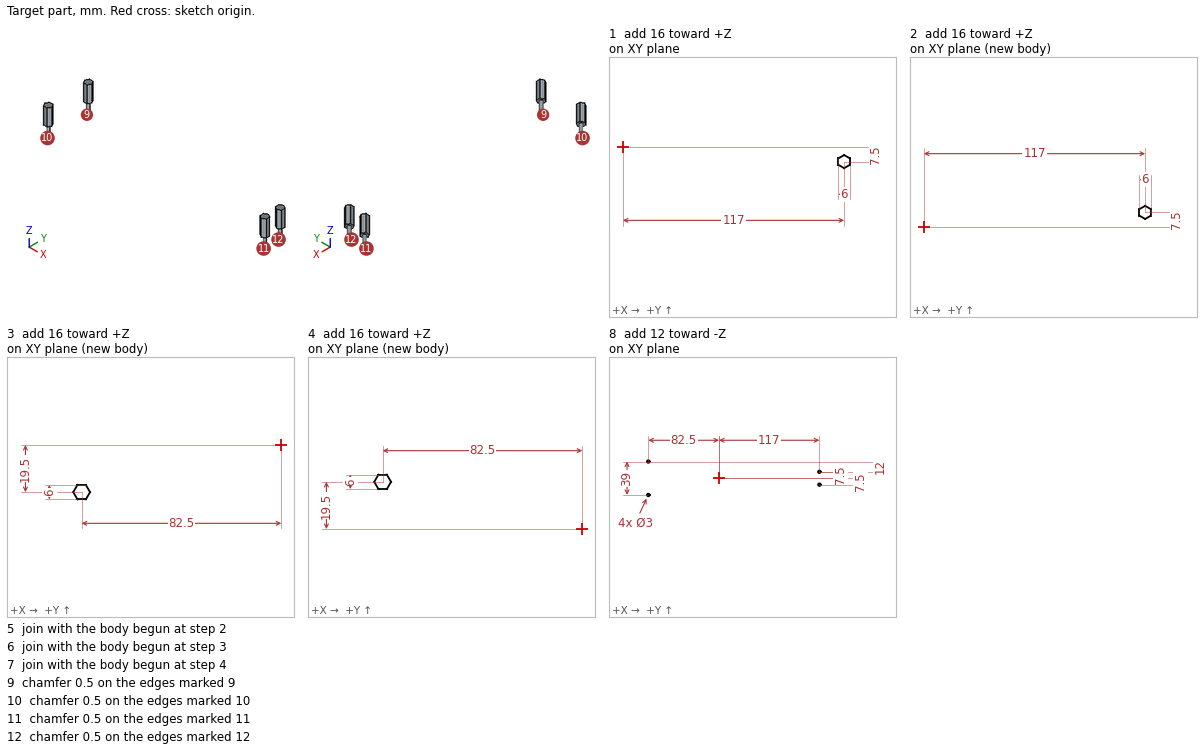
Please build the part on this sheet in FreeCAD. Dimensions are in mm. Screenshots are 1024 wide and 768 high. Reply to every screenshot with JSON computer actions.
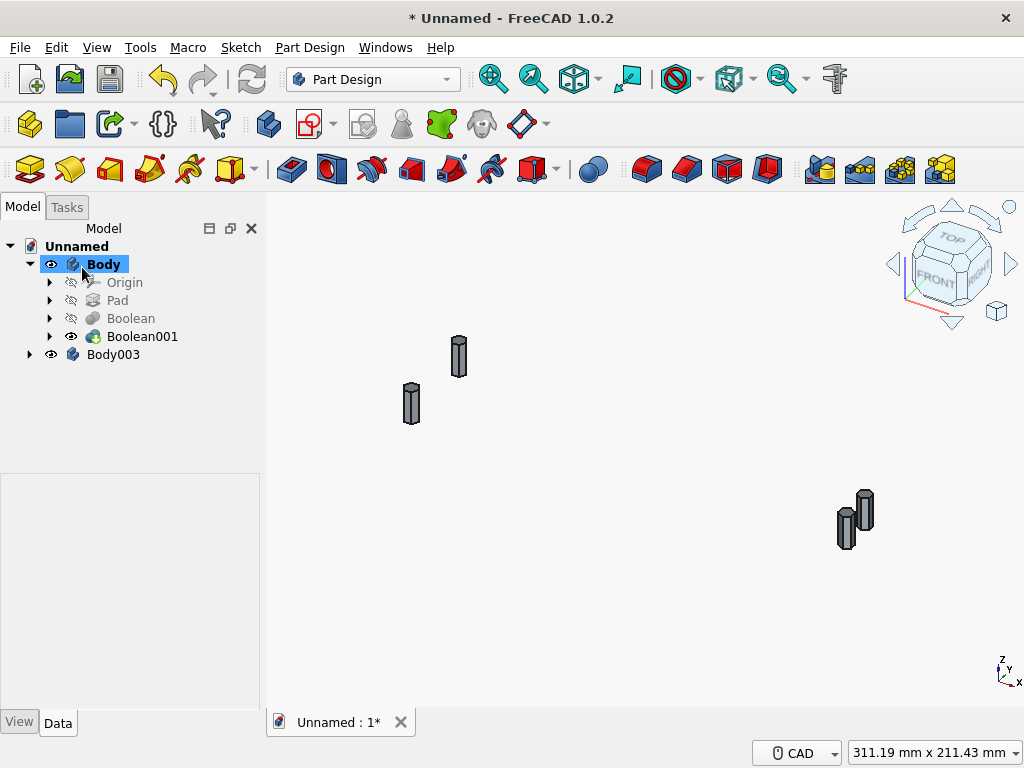
{"action": "left_click", "coordinate": [96, 354]}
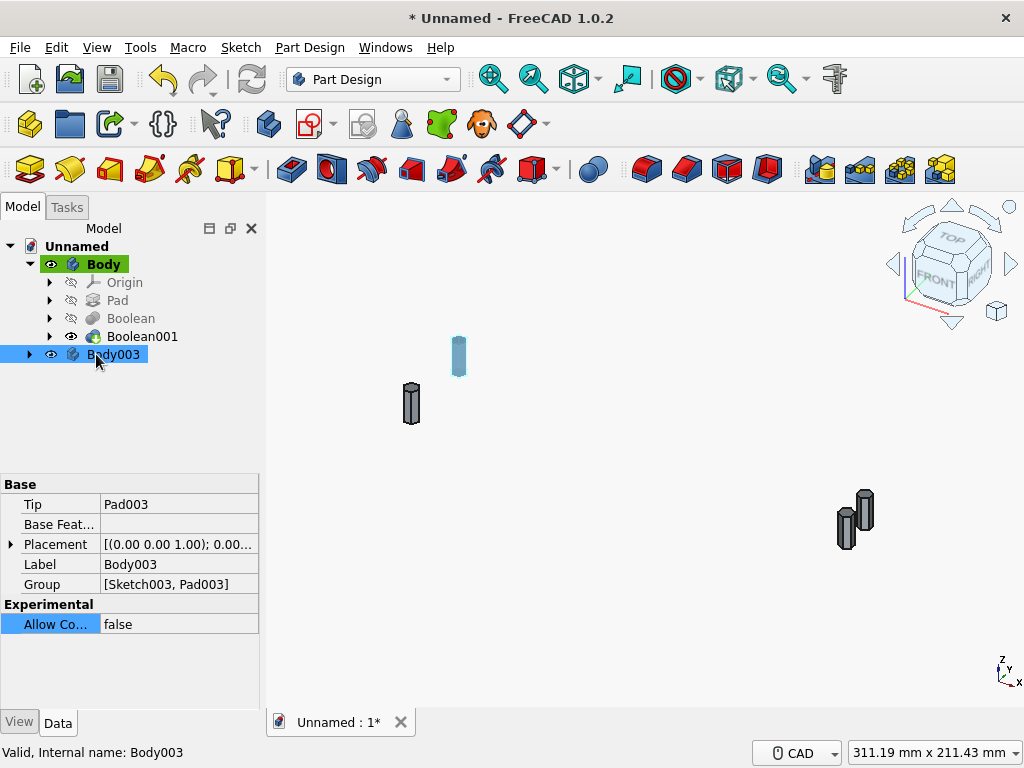
{"action": "left_click", "coordinate": [594, 170]}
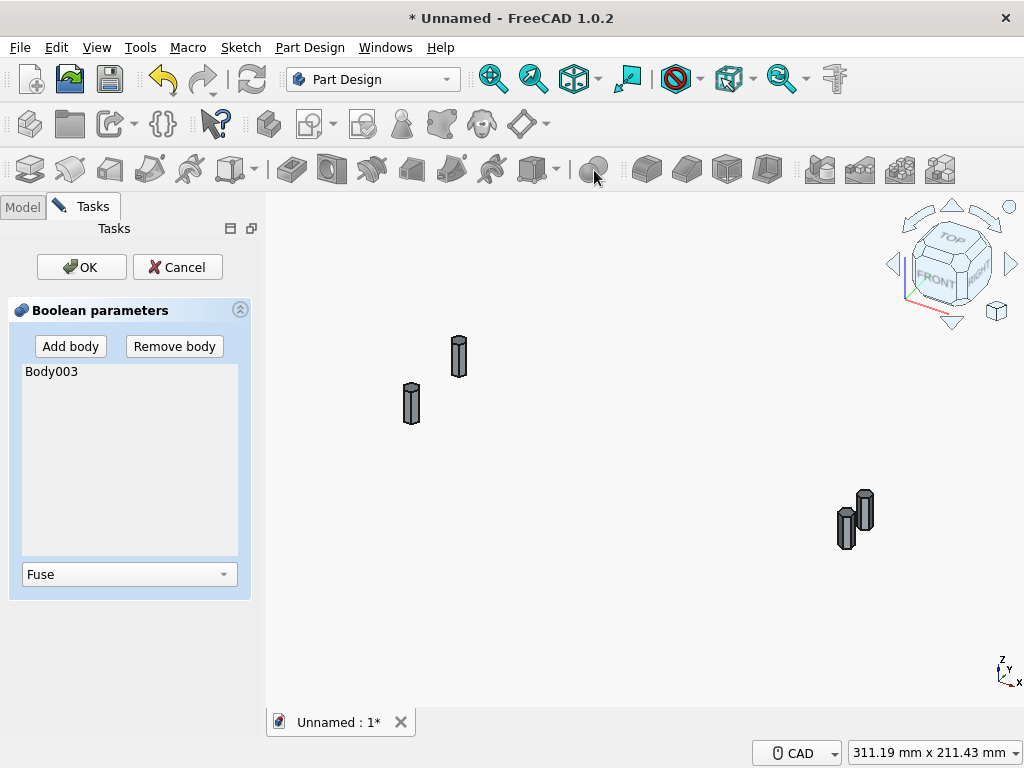
{"action": "left_click", "coordinate": [82, 267]}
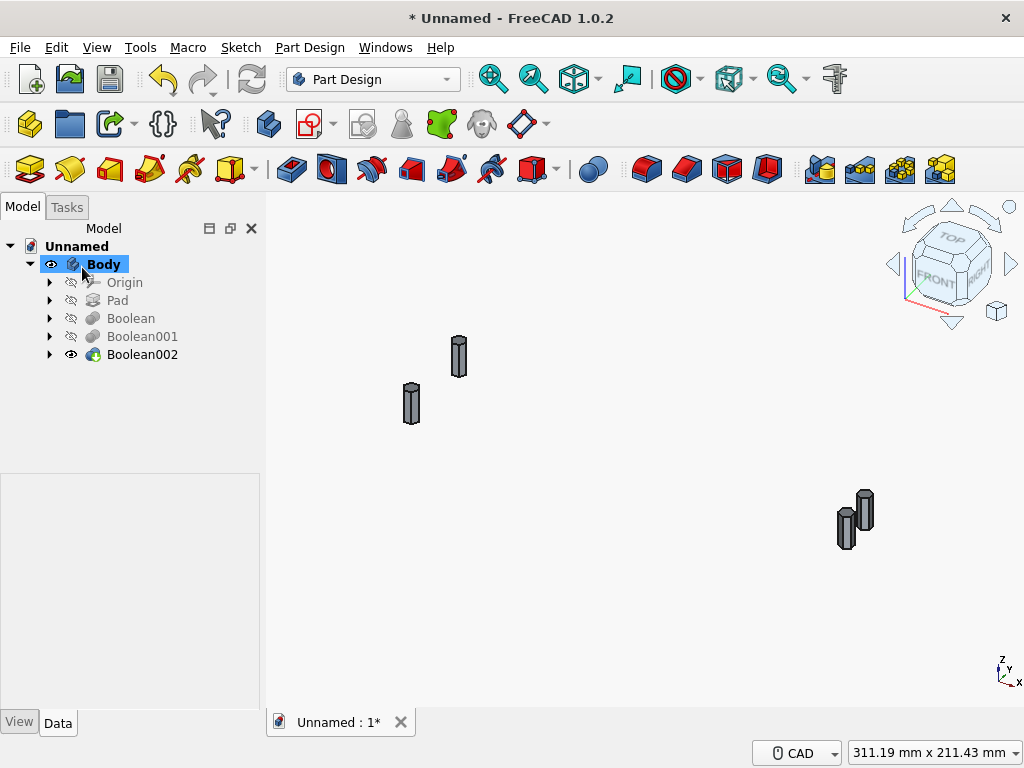
{"action": "key", "text": "5"}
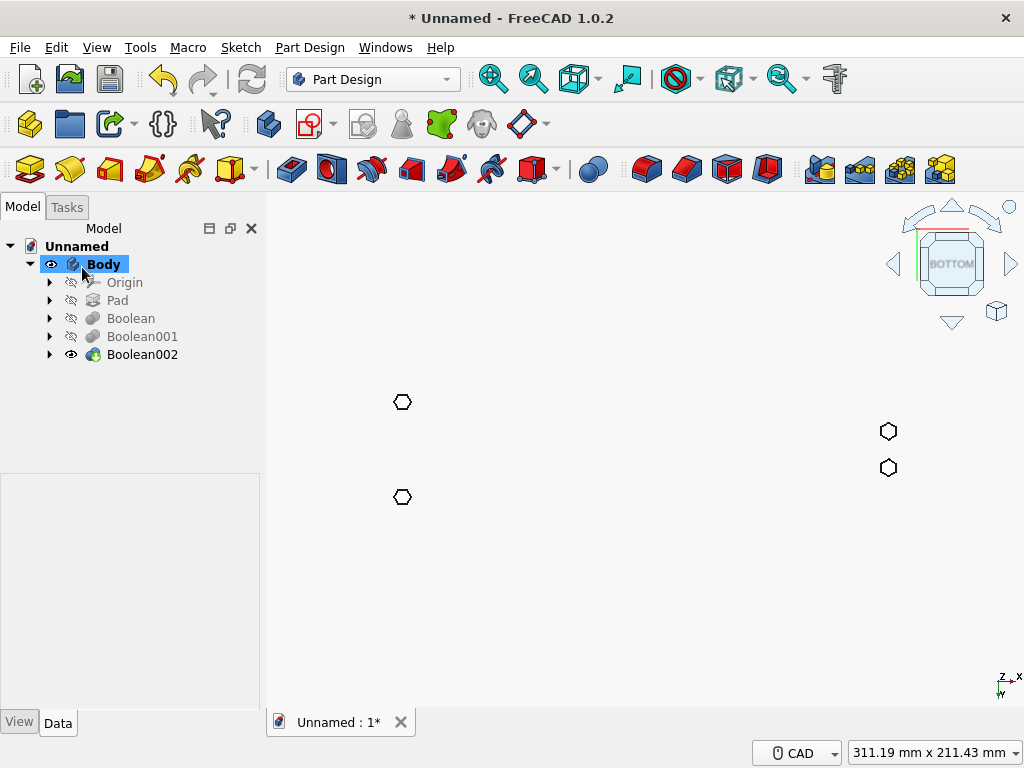
{"action": "key", "text": "1"}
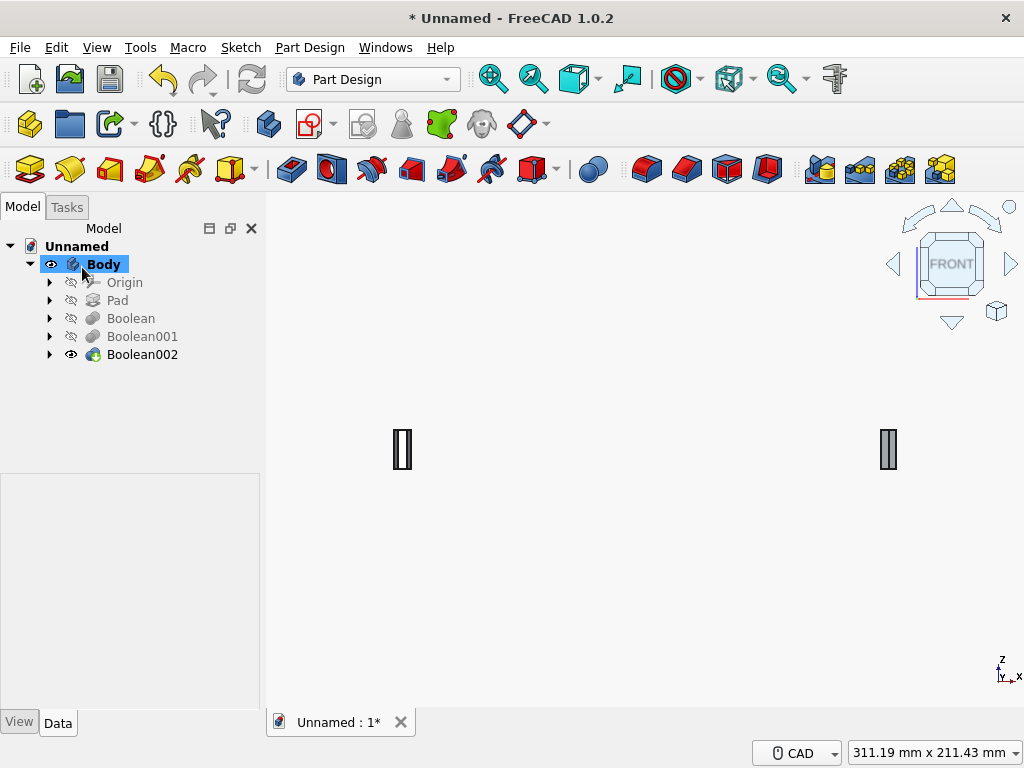
{"action": "key", "text": "3"}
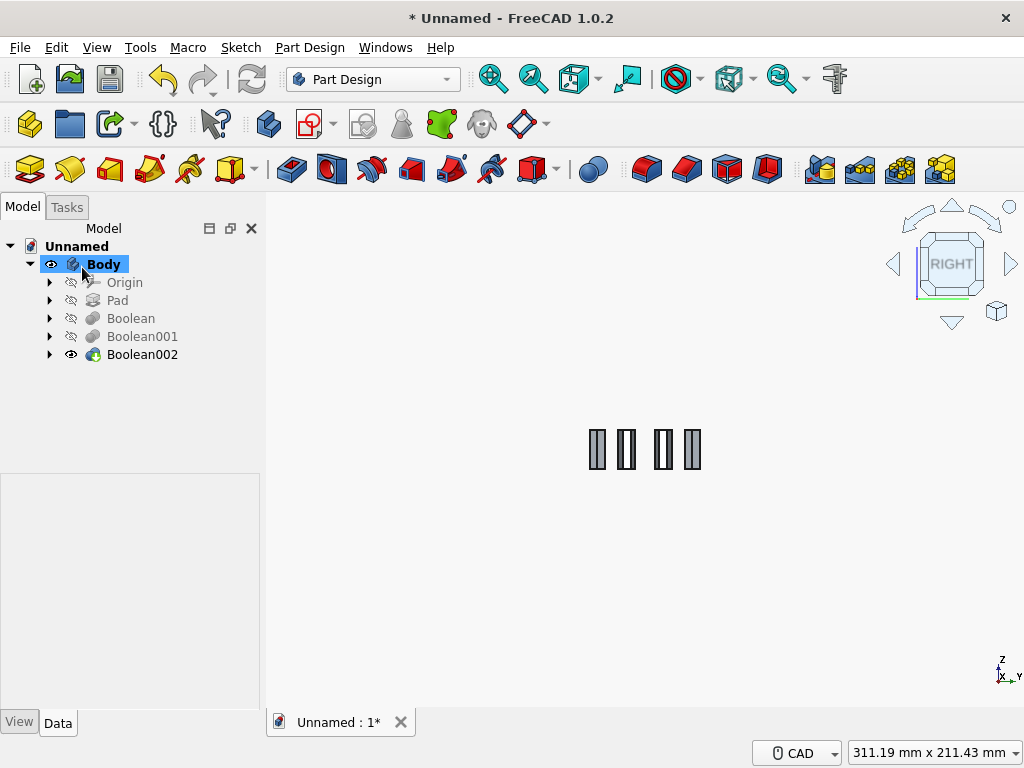
{"action": "left_click", "coordinate": [494, 80]}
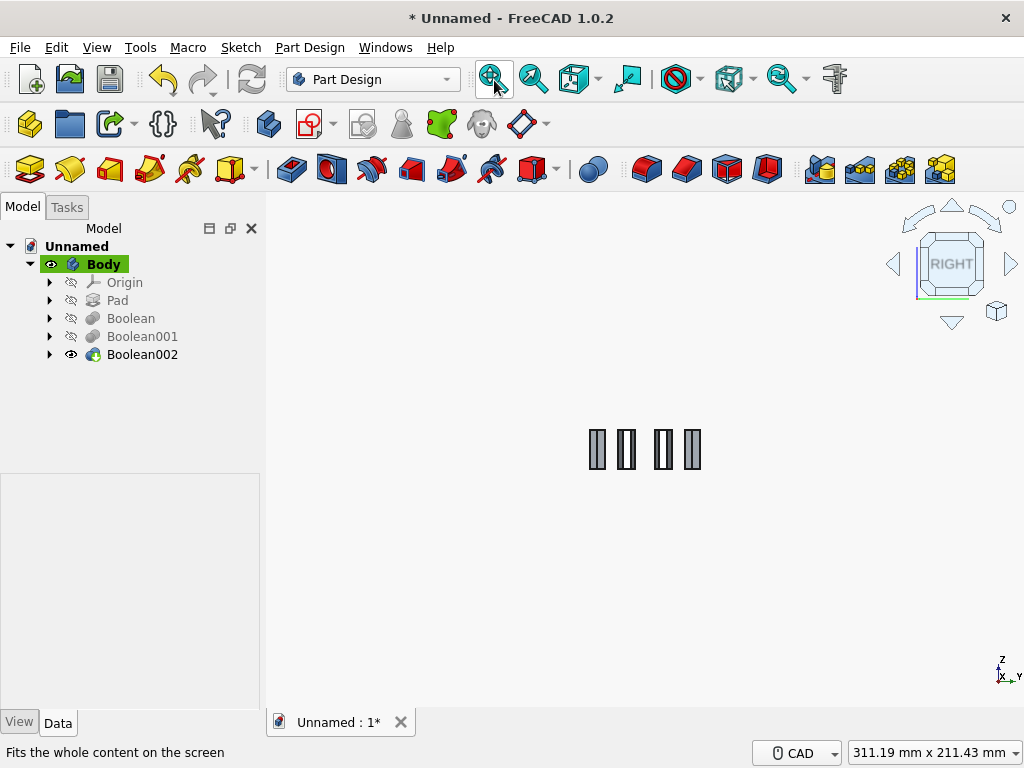
{"action": "left_click", "coordinate": [310, 124]}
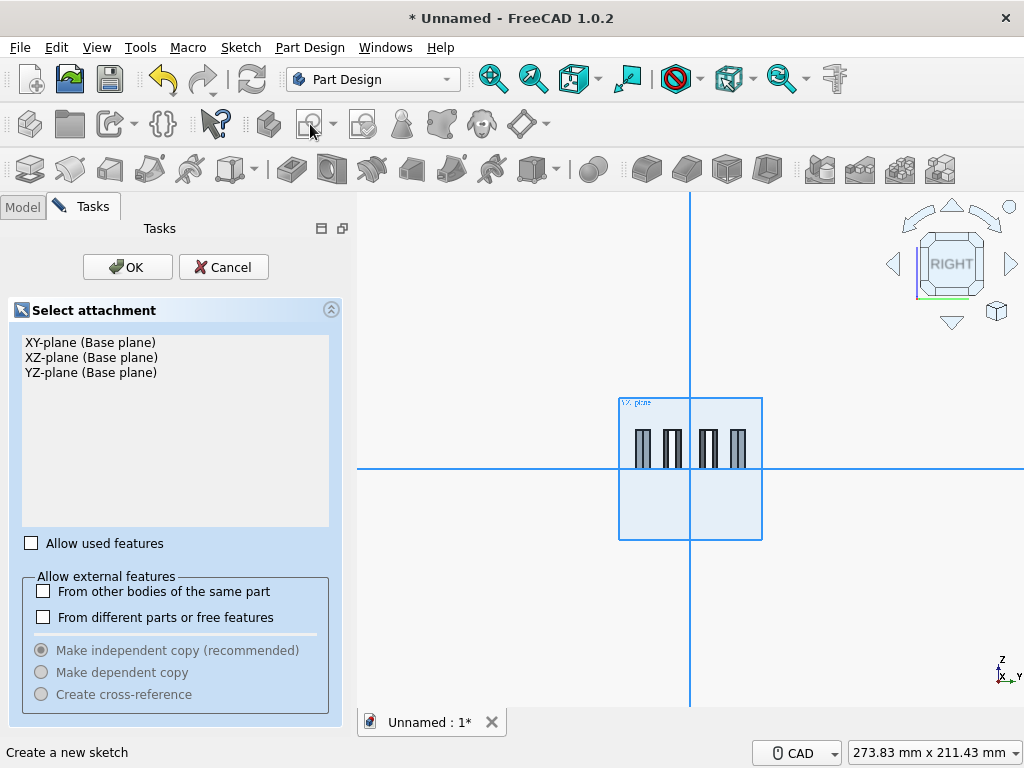
{"action": "left_click", "coordinate": [82, 342]}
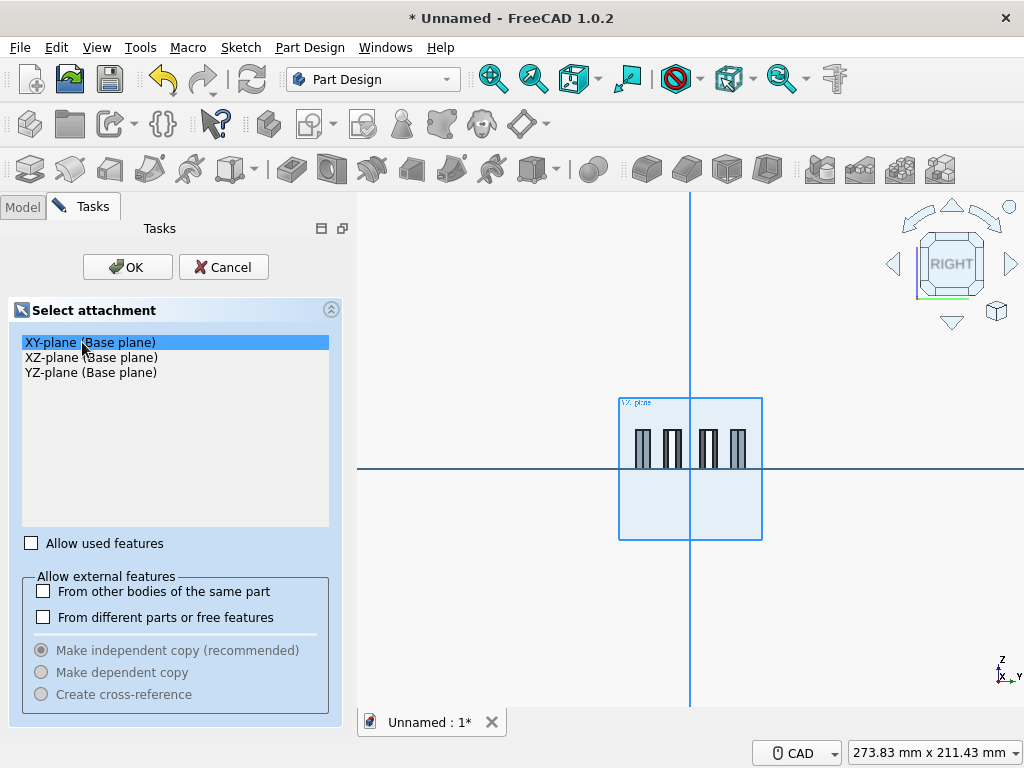
{"action": "left_click", "coordinate": [128, 267]}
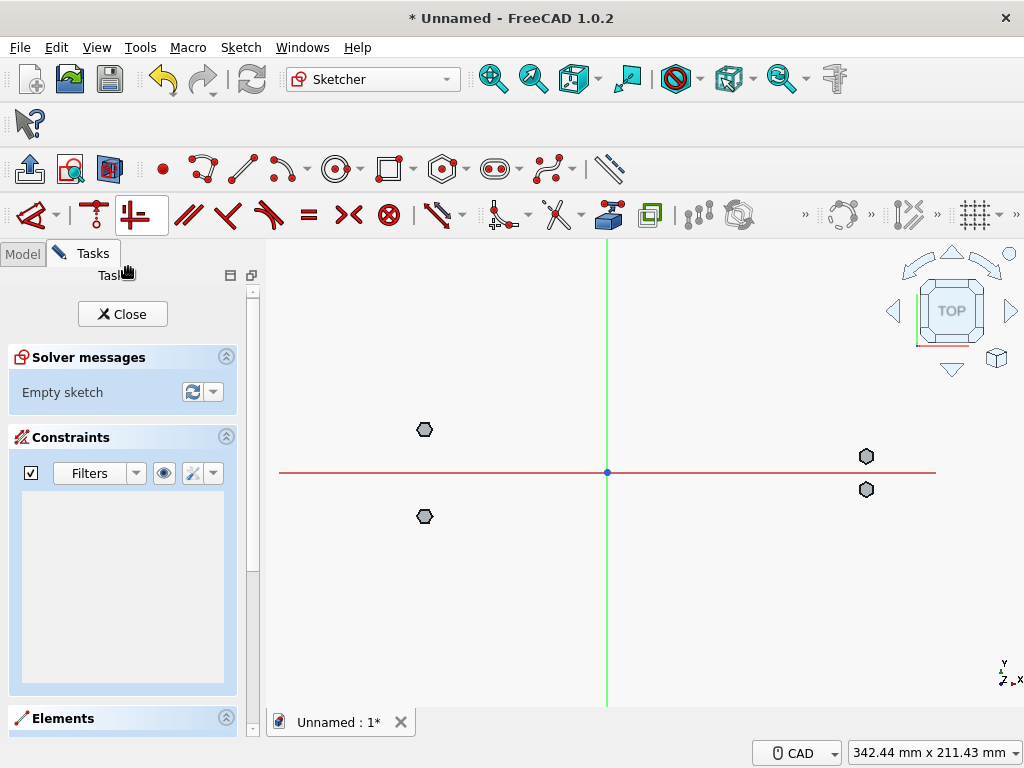
{"action": "left_click", "coordinate": [110, 170]}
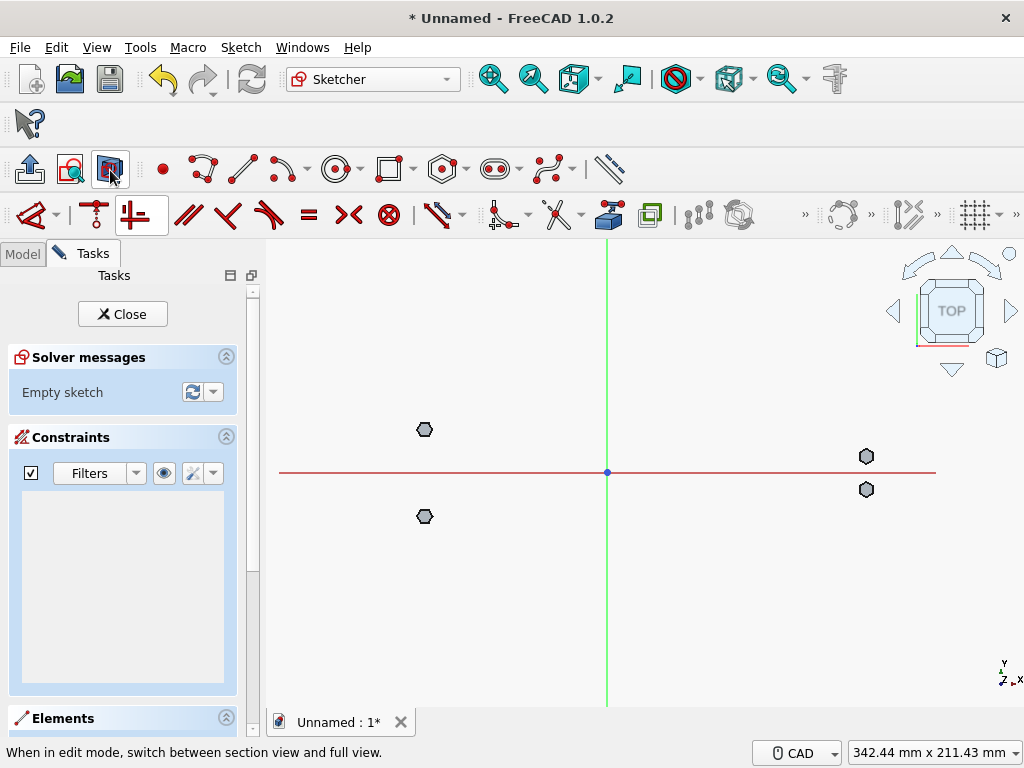
{"action": "scroll", "coordinate": [294, 473], "scroll_direction": "down", "scroll_amount": 1}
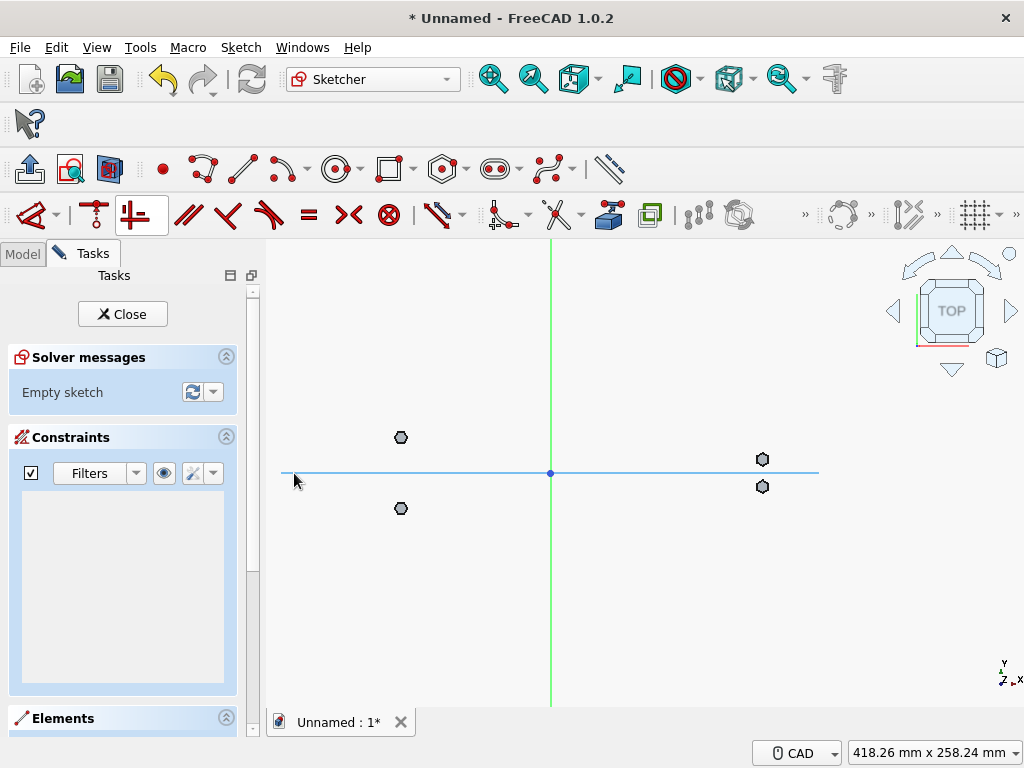
{"action": "left_click", "coordinate": [336, 170]}